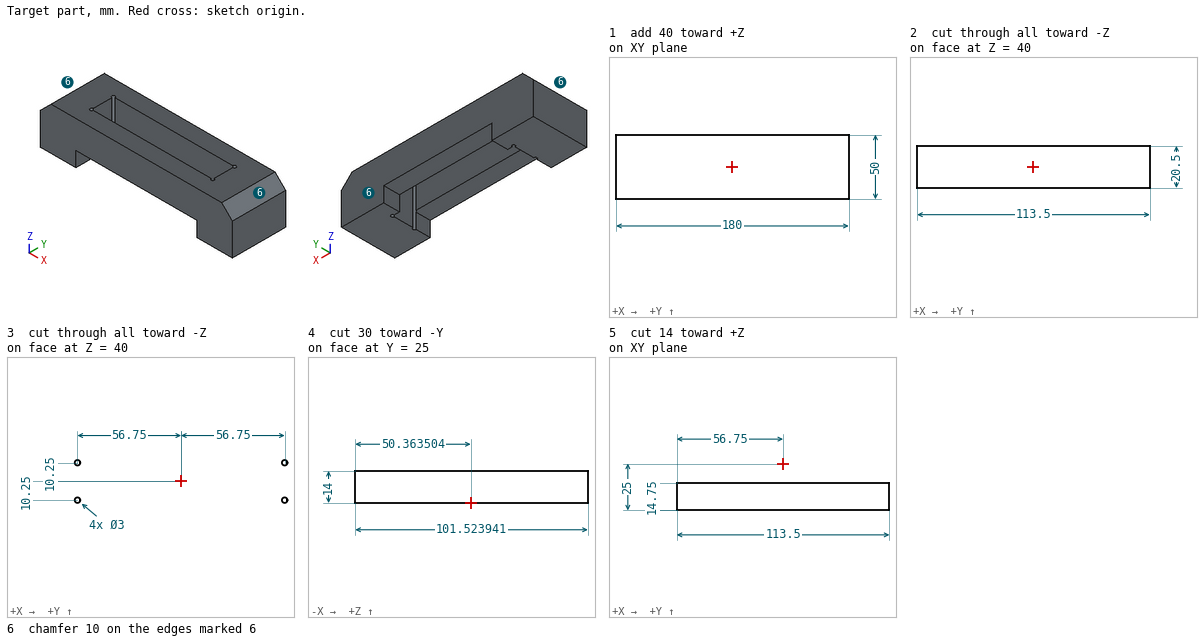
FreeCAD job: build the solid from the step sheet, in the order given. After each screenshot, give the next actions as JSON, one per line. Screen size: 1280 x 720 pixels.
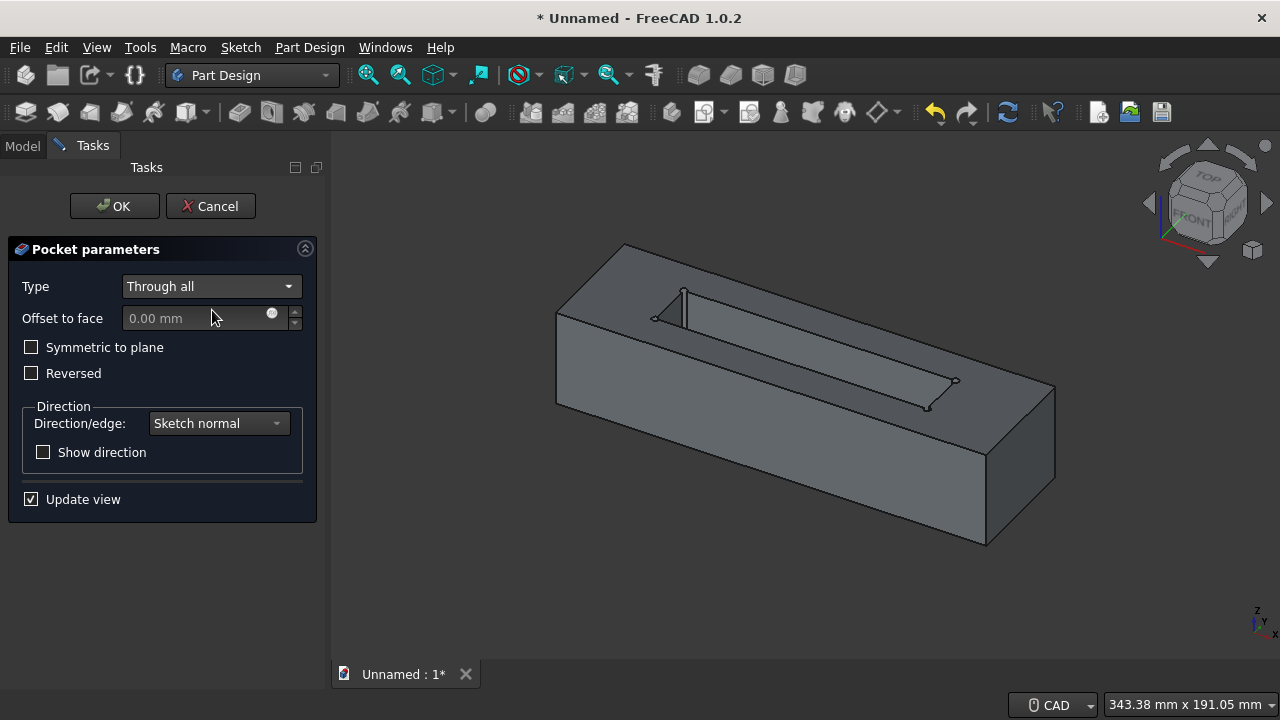
{"action": "left_click", "coordinate": [115, 206]}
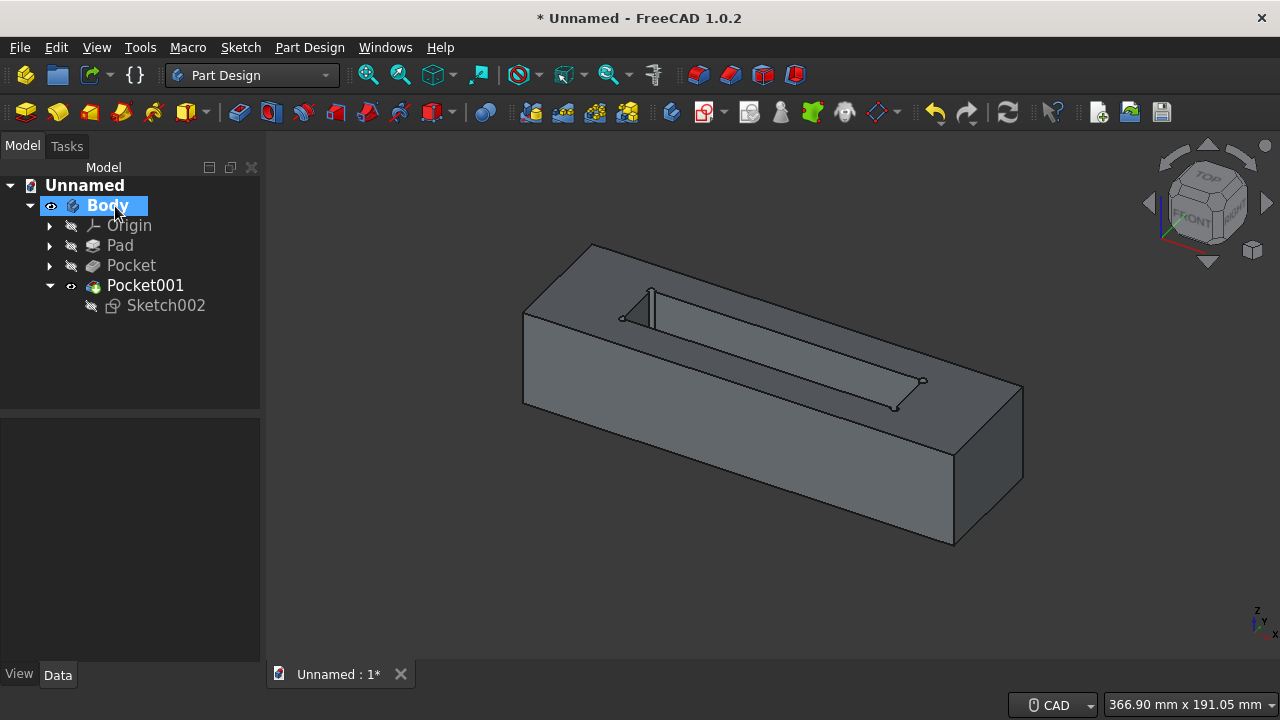
{"action": "key", "text": "4"}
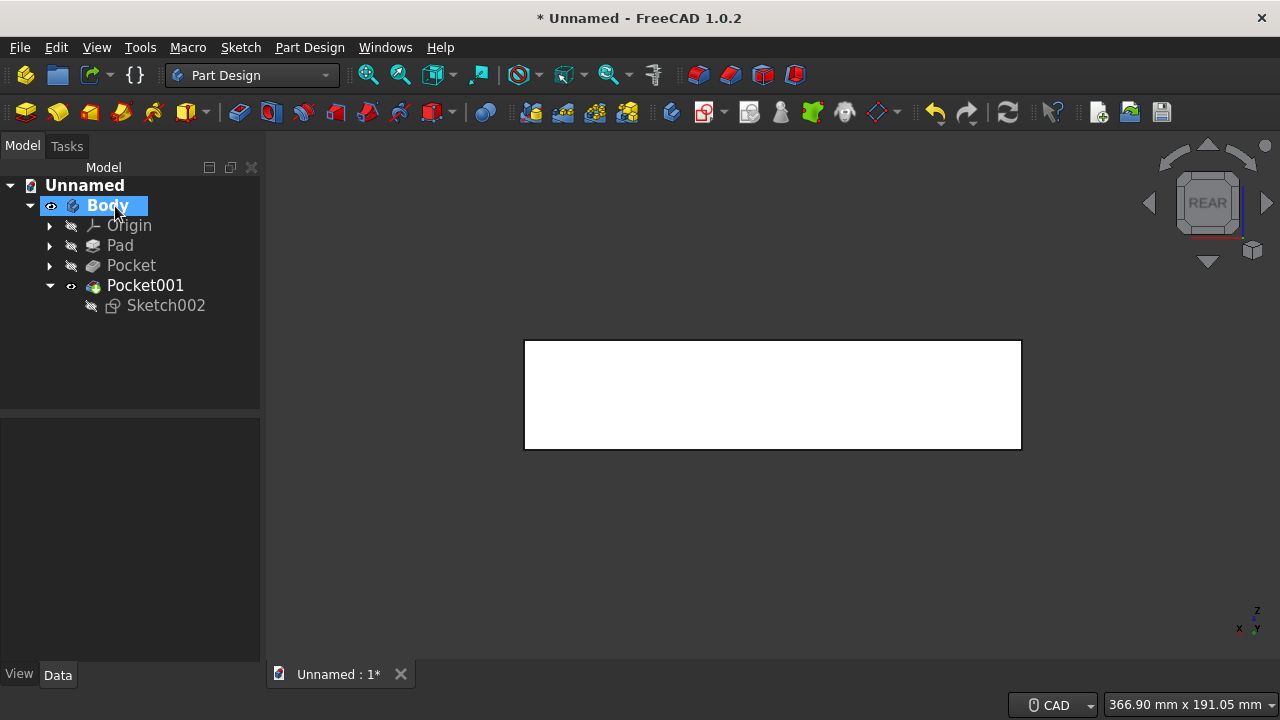
{"action": "left_click", "coordinate": [631, 394]}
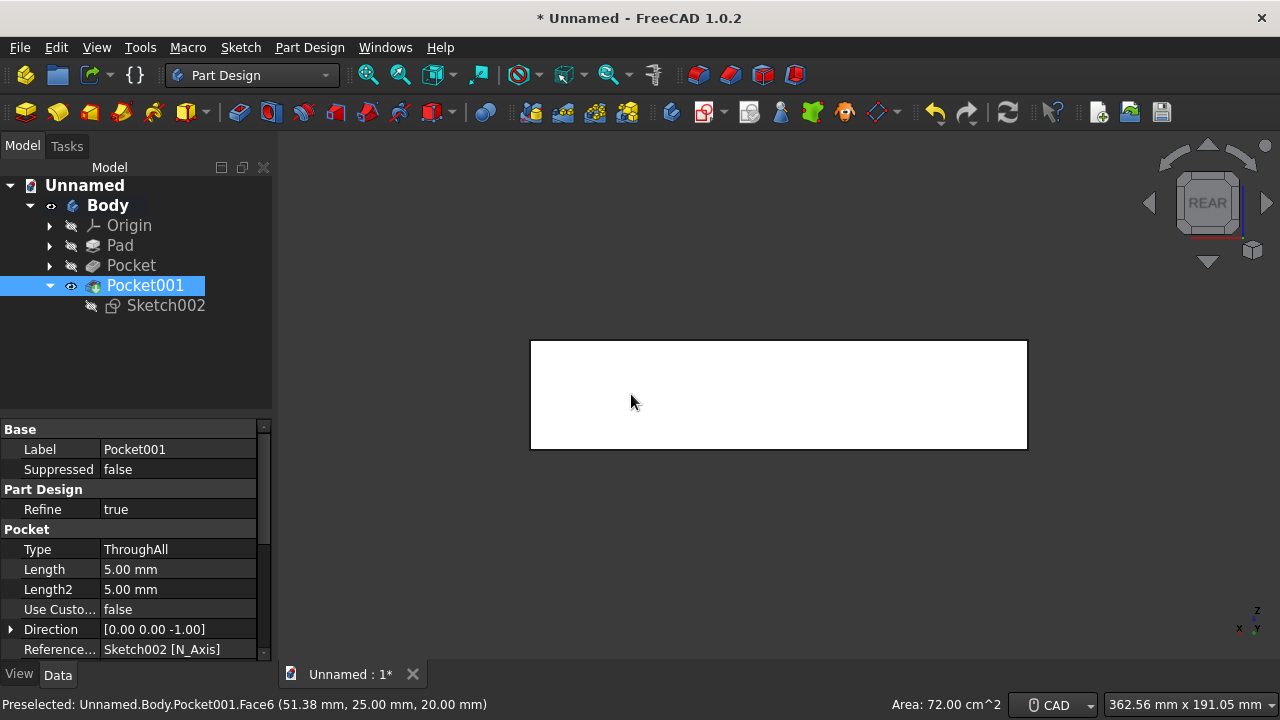
{"action": "left_click", "coordinate": [704, 112]}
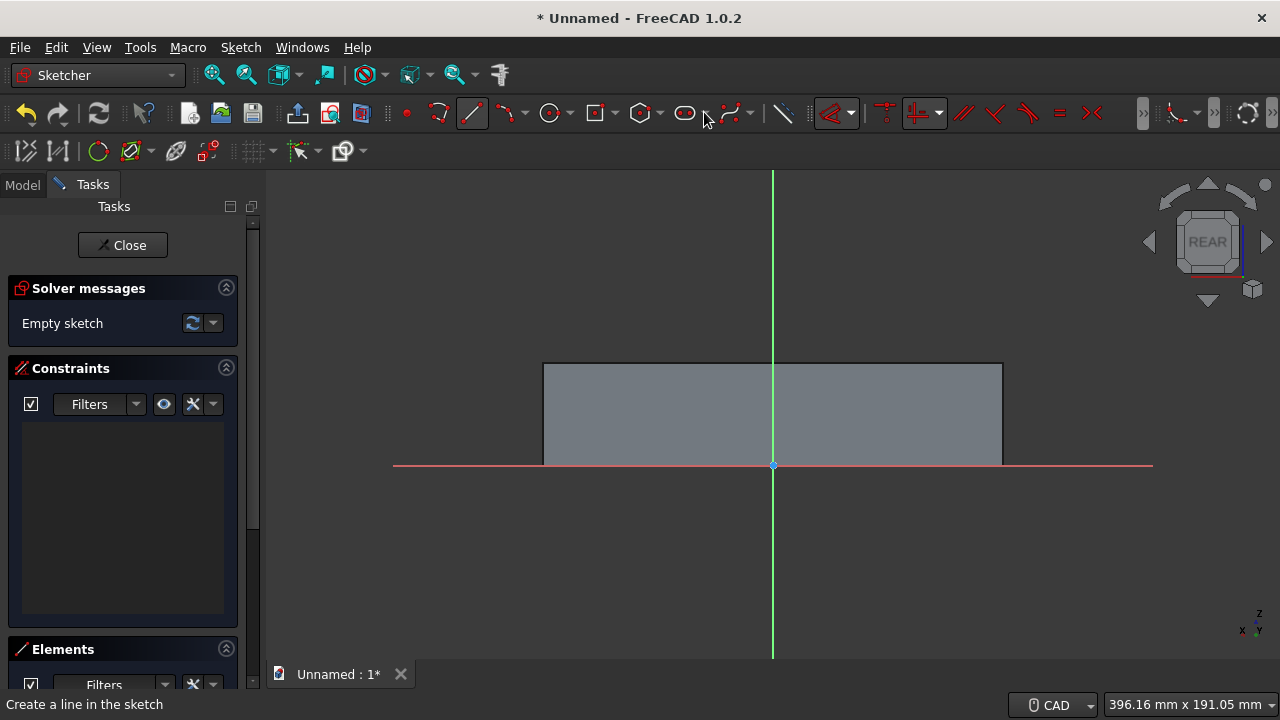
{"action": "scroll", "coordinate": [831, 475], "scroll_direction": "up", "scroll_amount": 4}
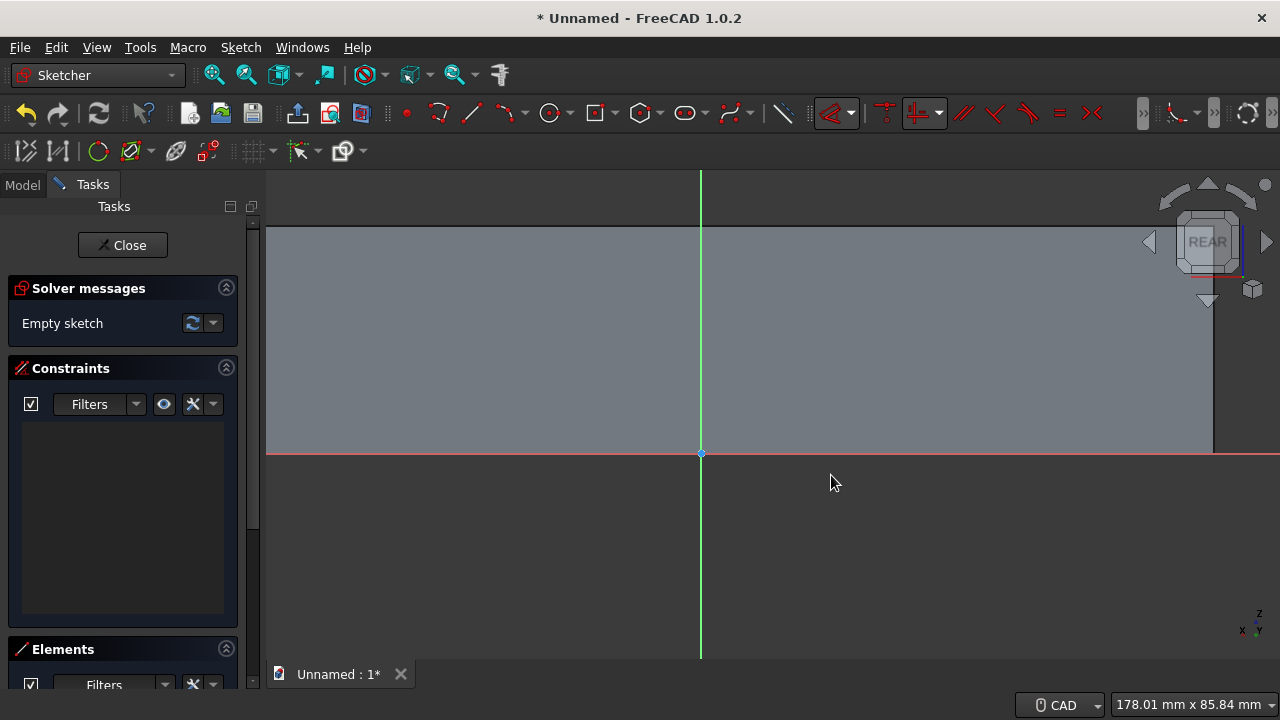
{"action": "left_click", "coordinate": [618, 114]}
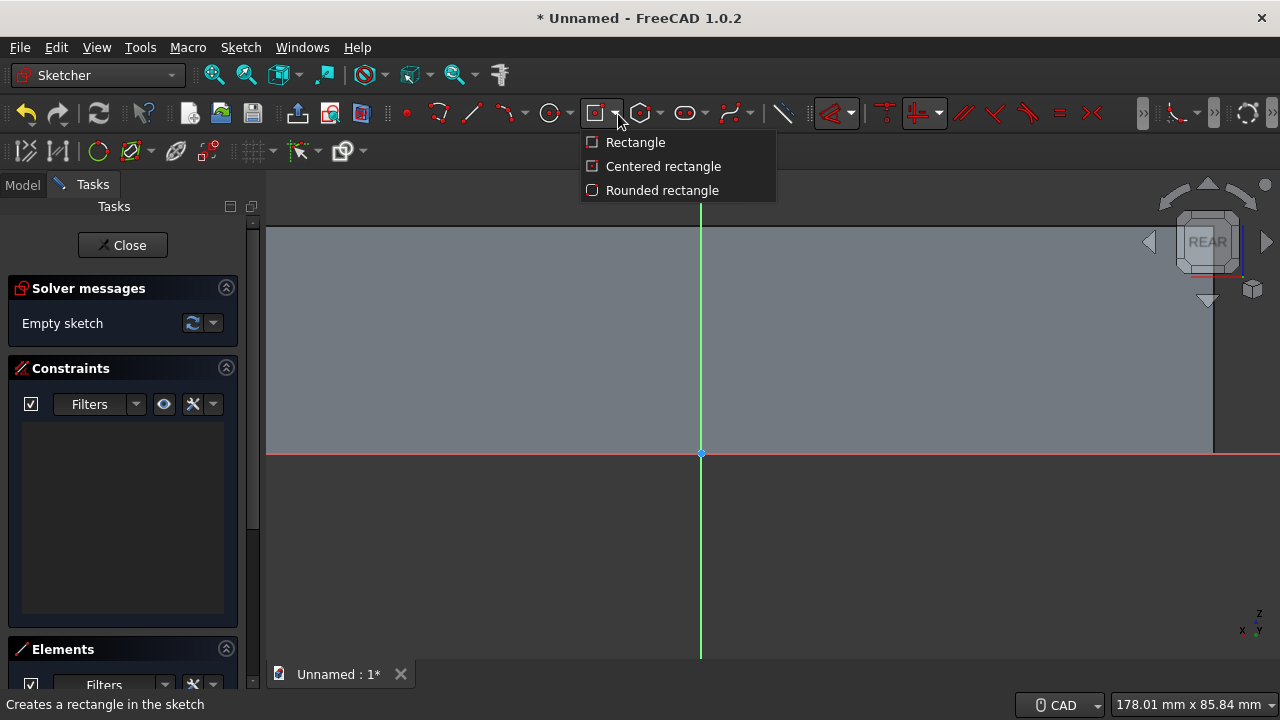
{"action": "left_click", "coordinate": [678, 142]}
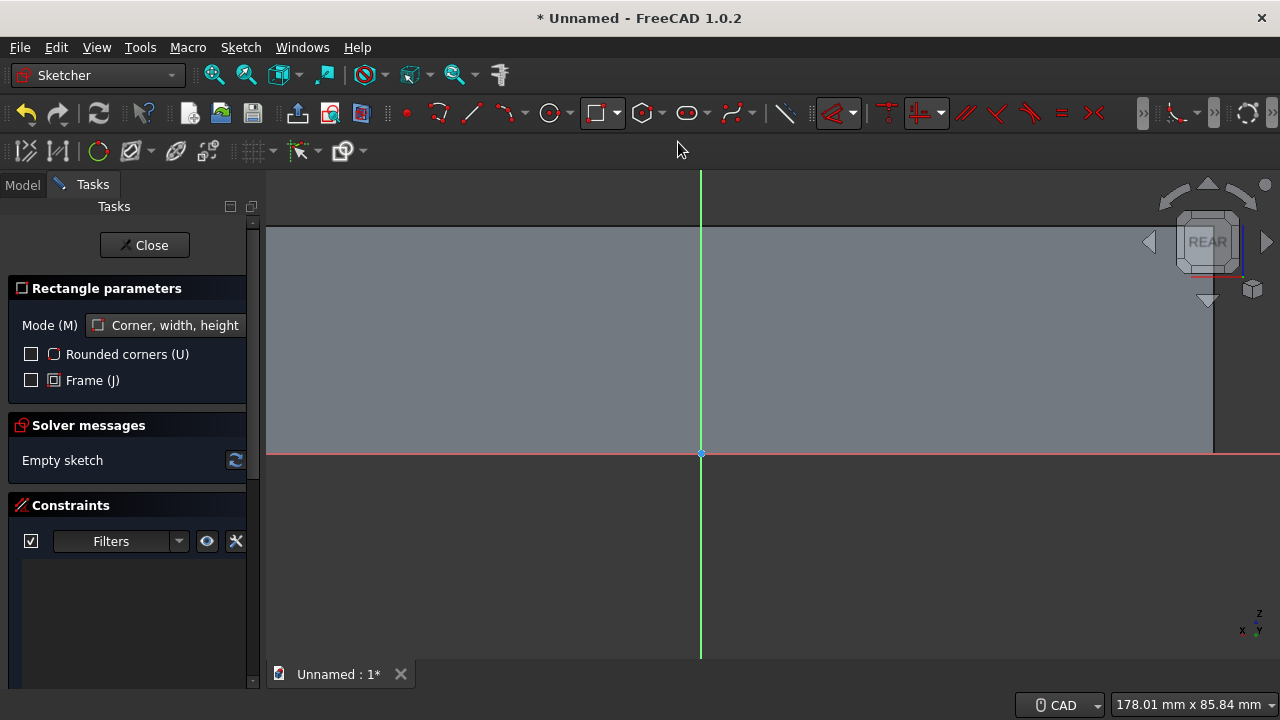
{"action": "left_click", "coordinate": [414, 374]}
{"action": "left_click", "coordinate": [993, 454]}
{"action": "key", "text": "Escape"}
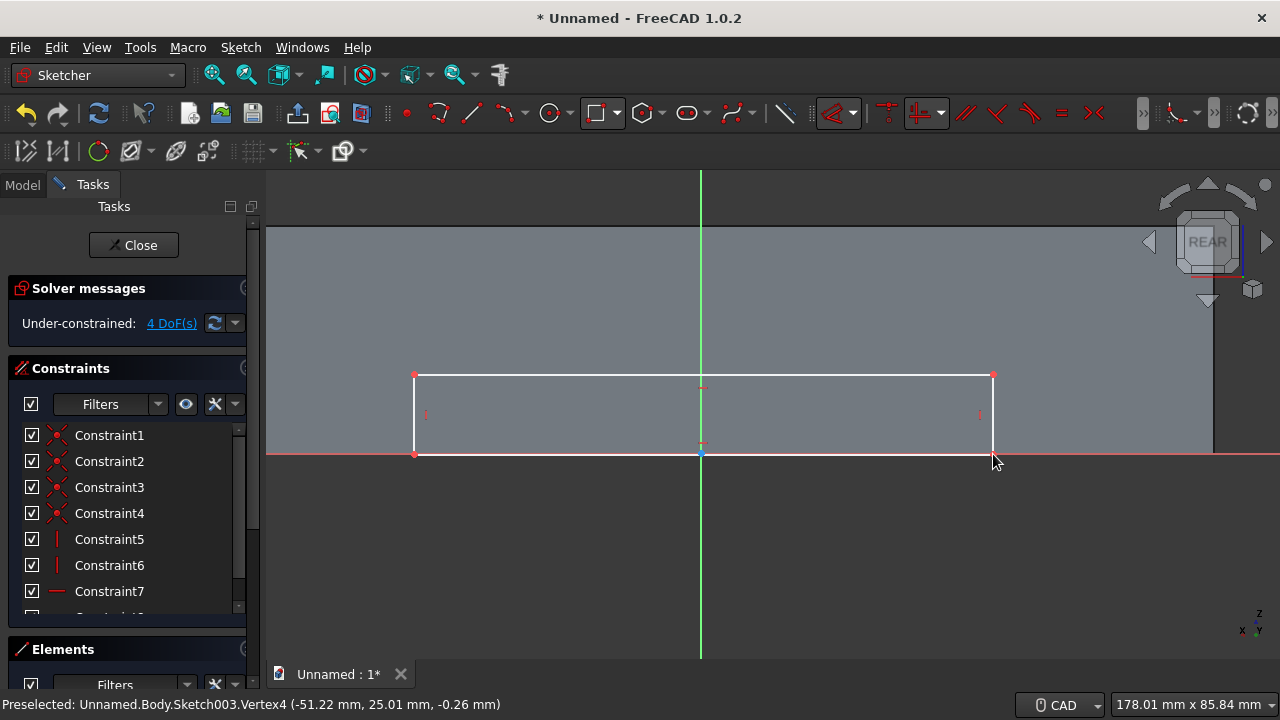
{"action": "left_click", "coordinate": [414, 455]}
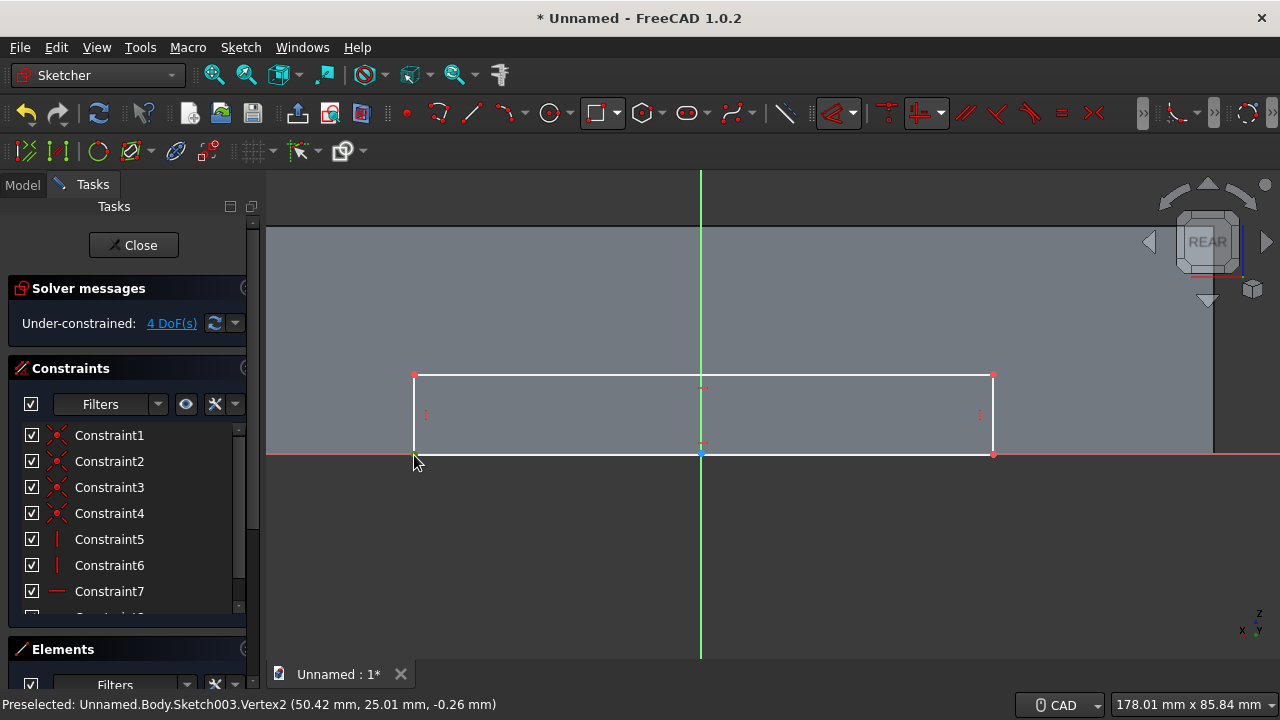
{"action": "left_click", "coordinate": [353, 454]}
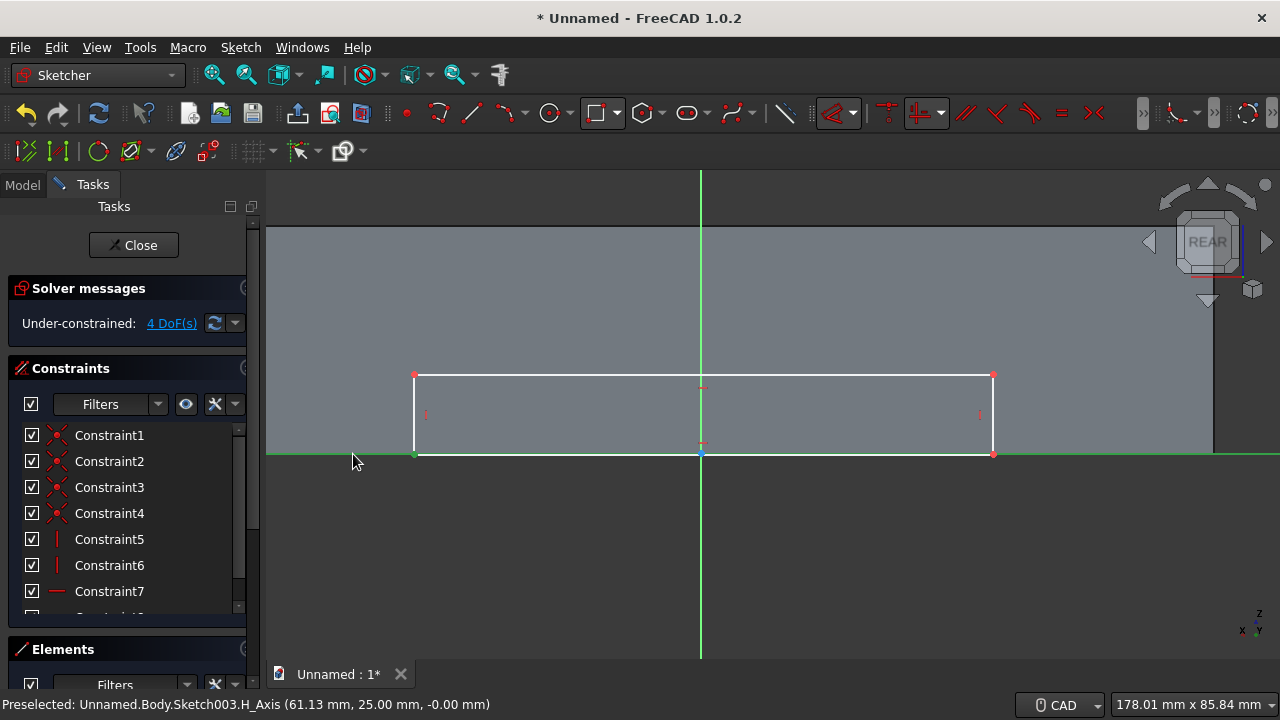
{"action": "left_click", "coordinate": [888, 114]}